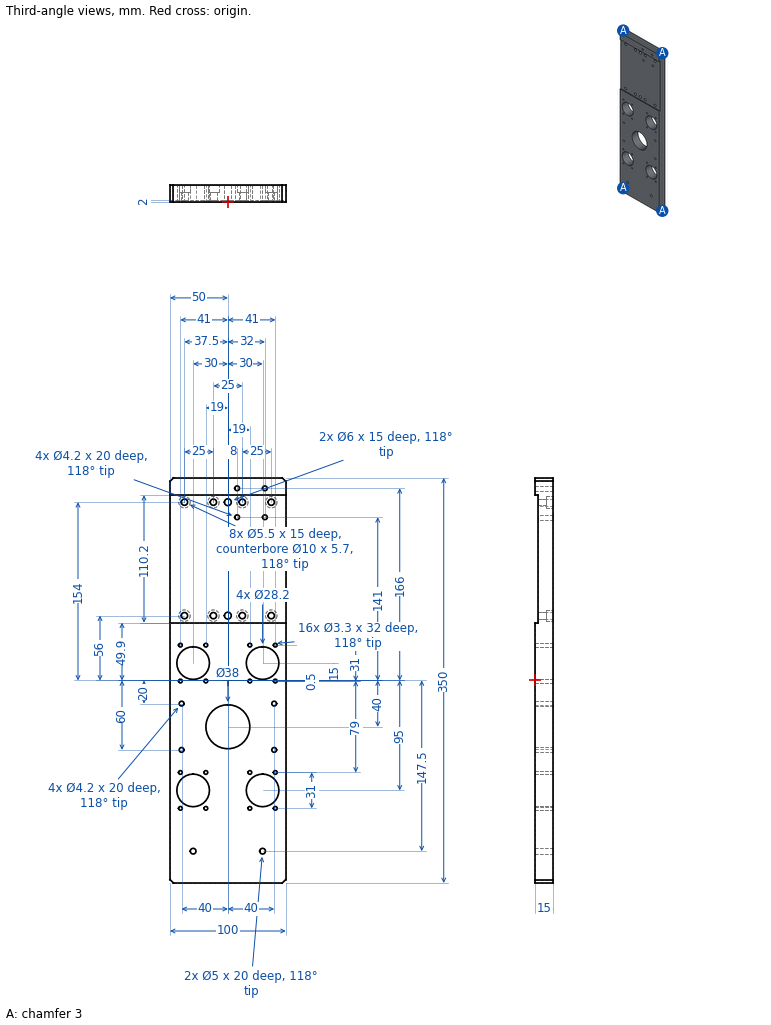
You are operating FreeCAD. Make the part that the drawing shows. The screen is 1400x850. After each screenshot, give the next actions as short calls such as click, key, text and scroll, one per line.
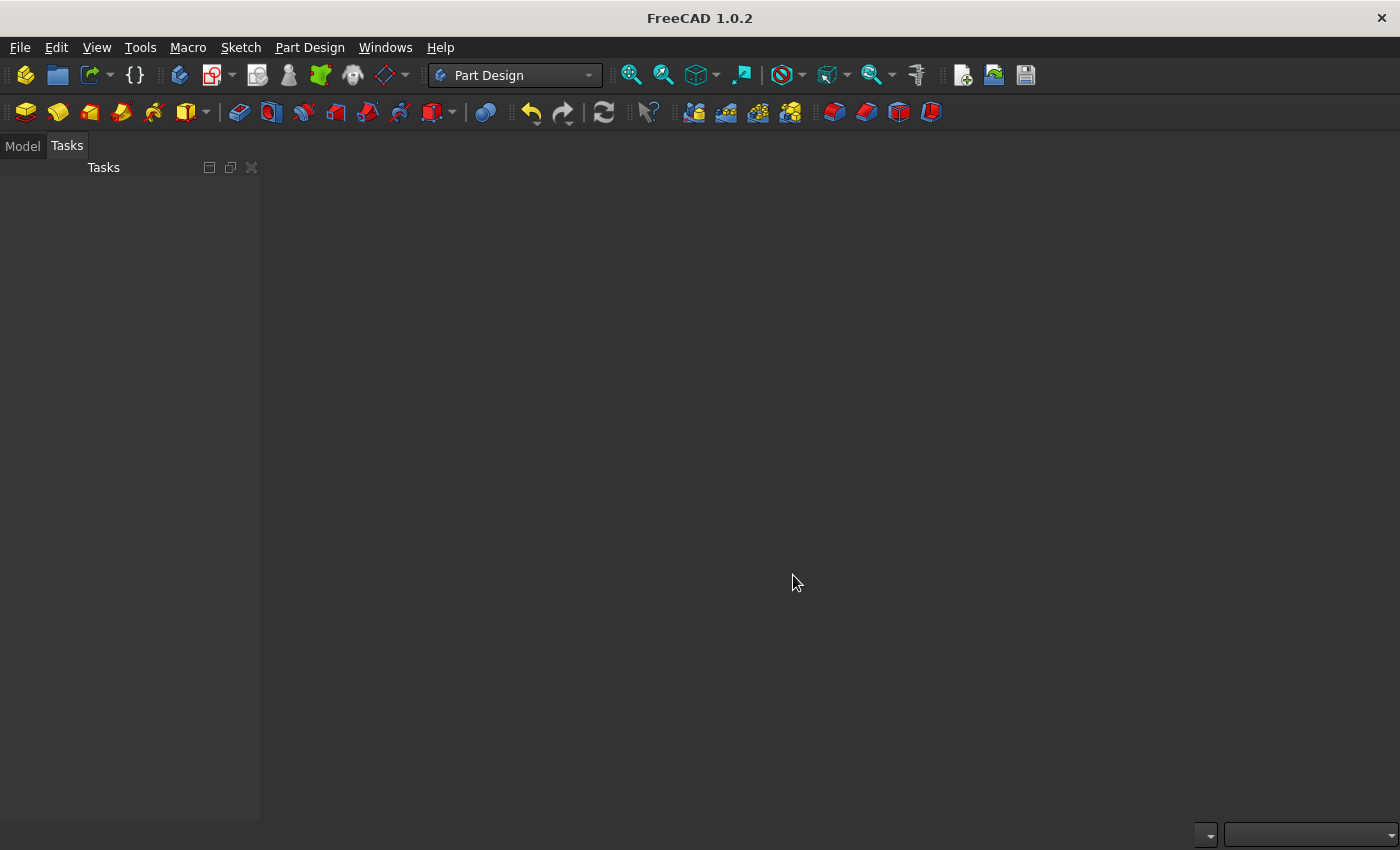
key(ctrl+n)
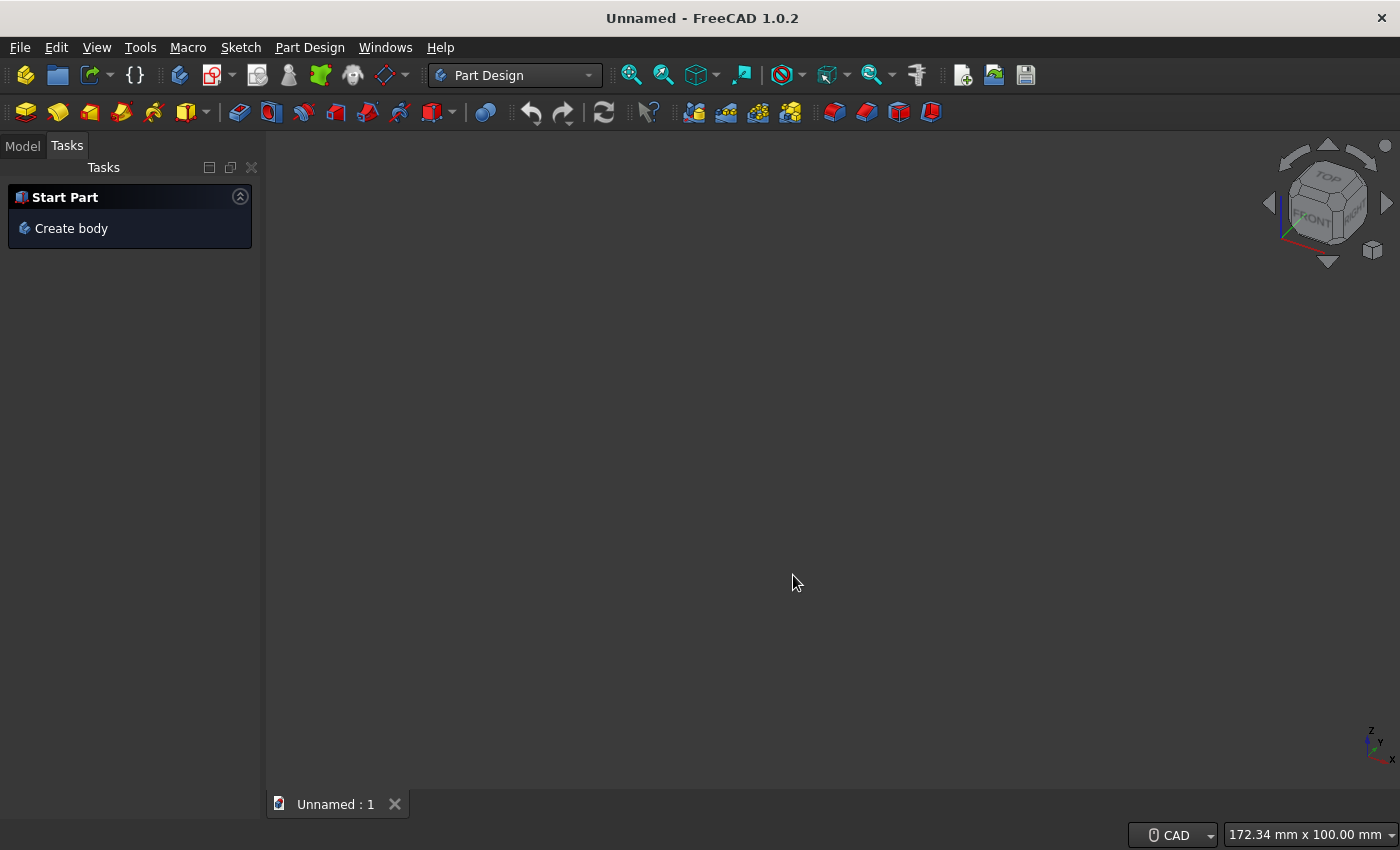
click(212, 76)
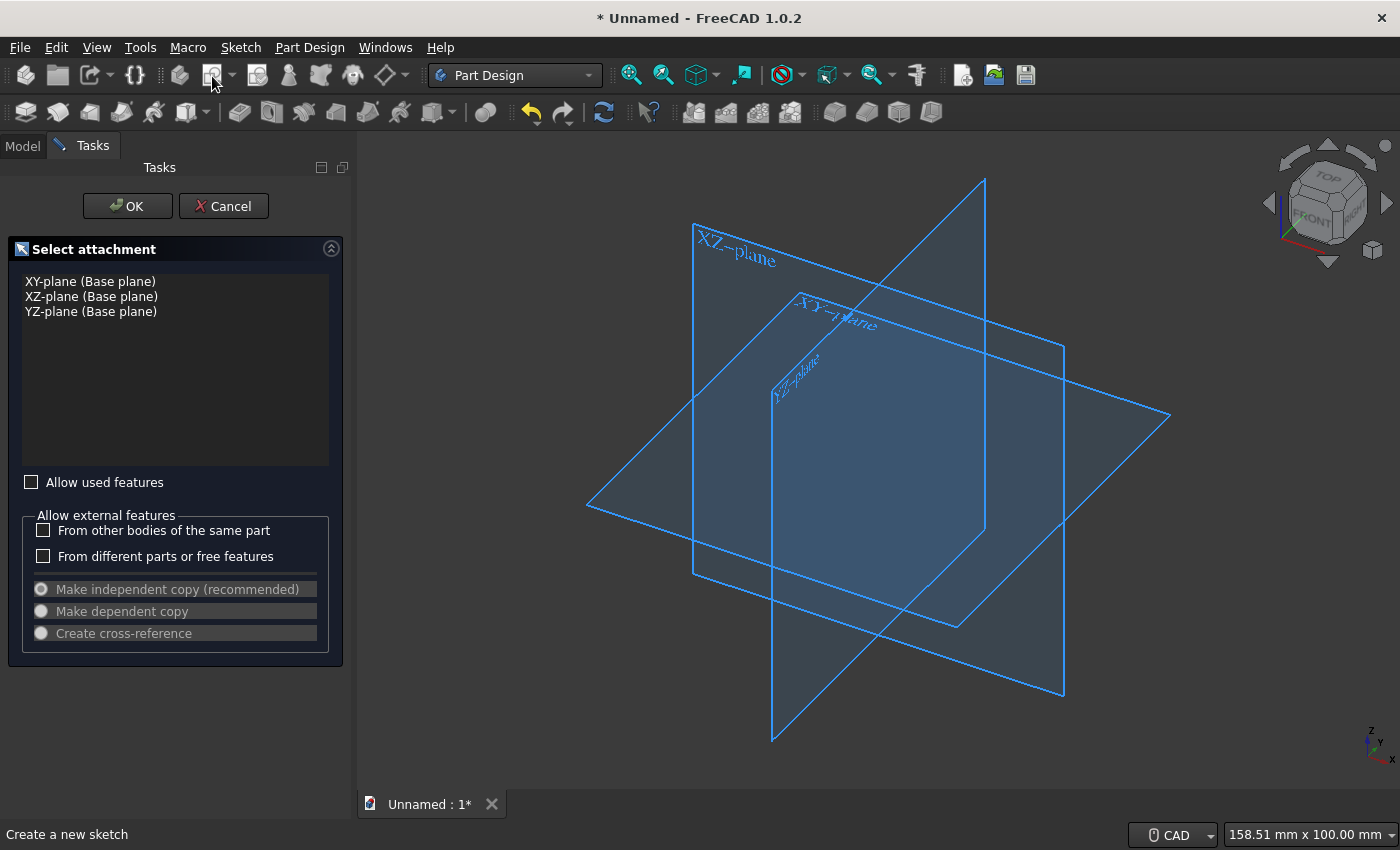
click(82, 296)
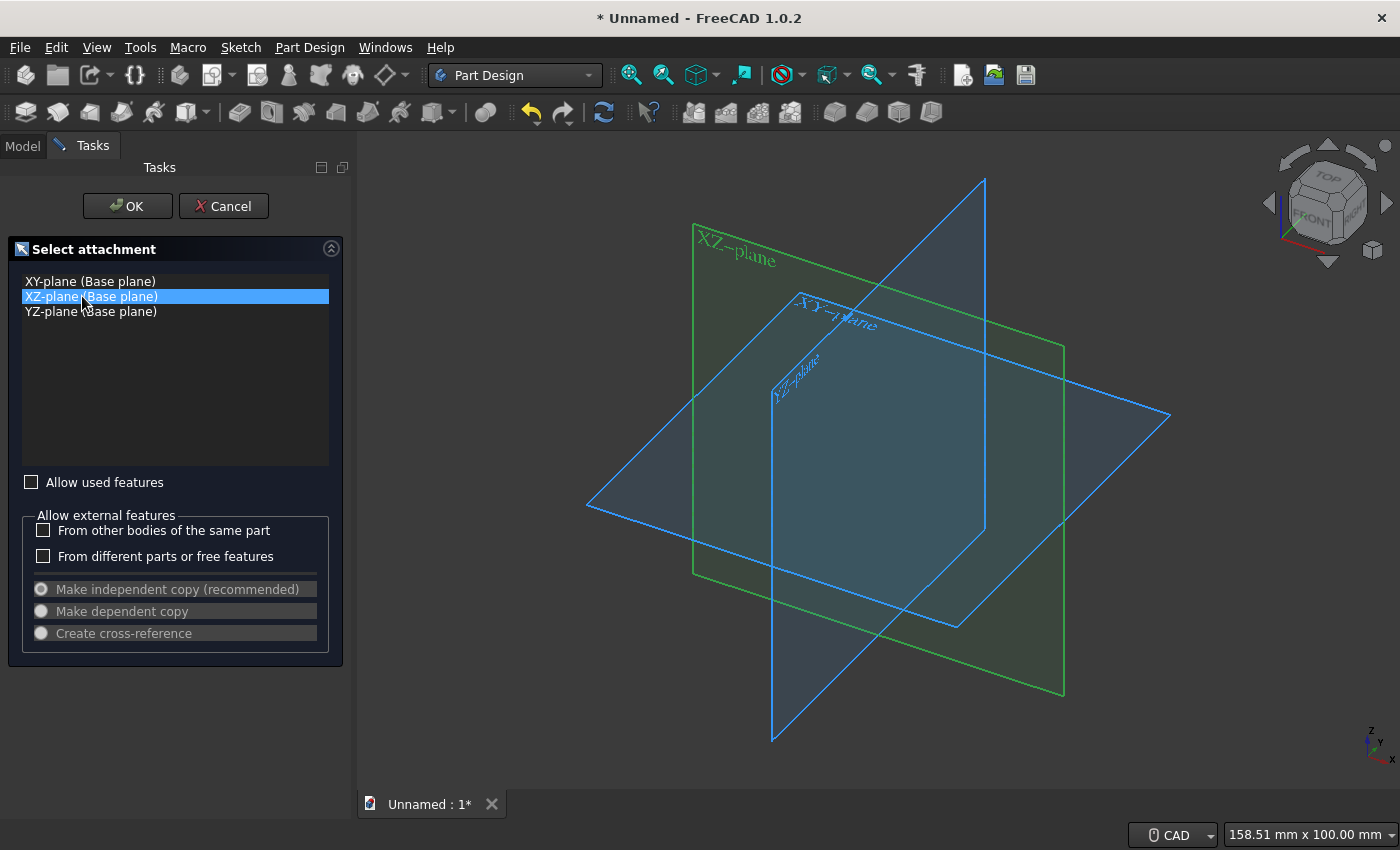
click(128, 206)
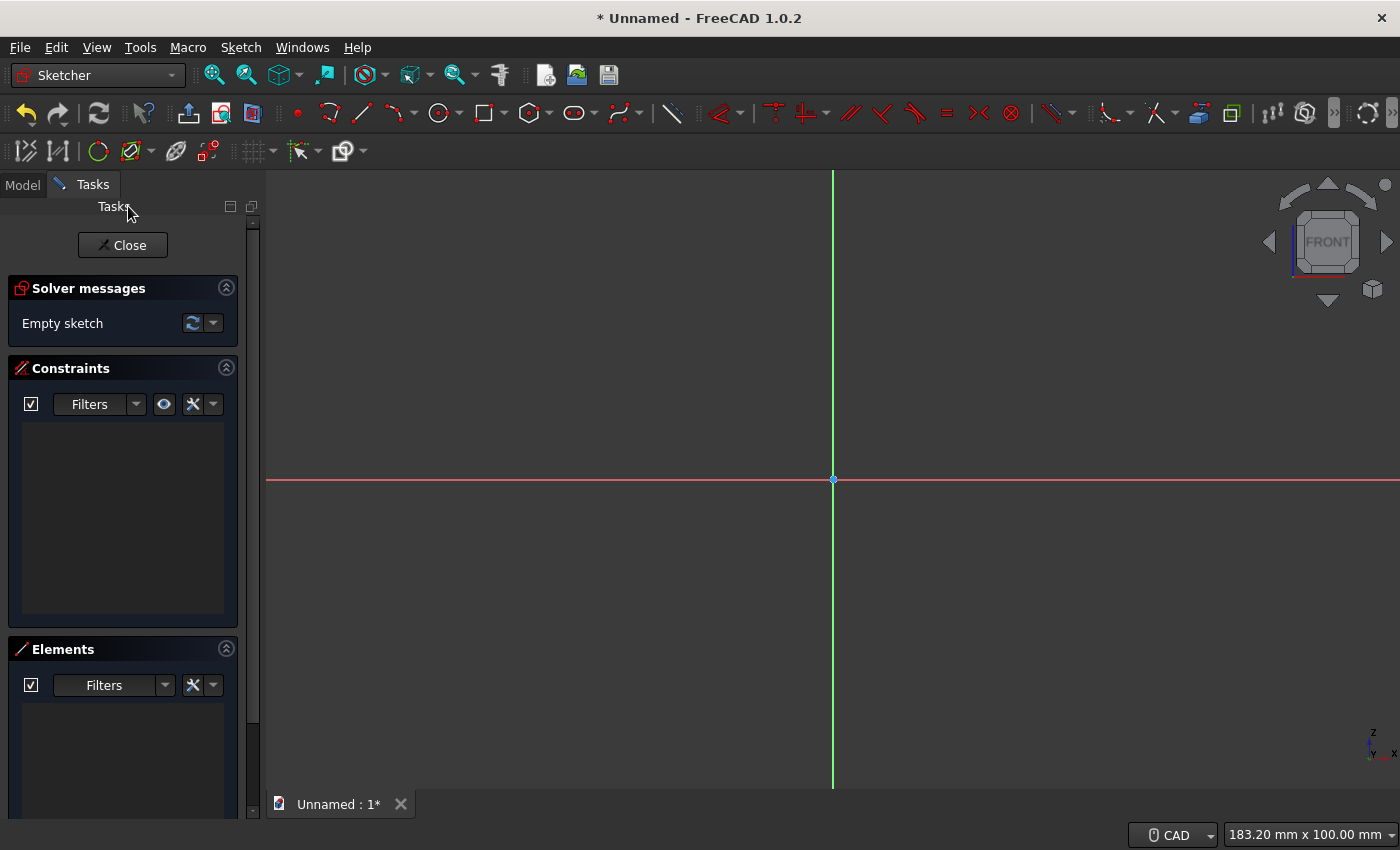
scroll(747, 480, down, 8)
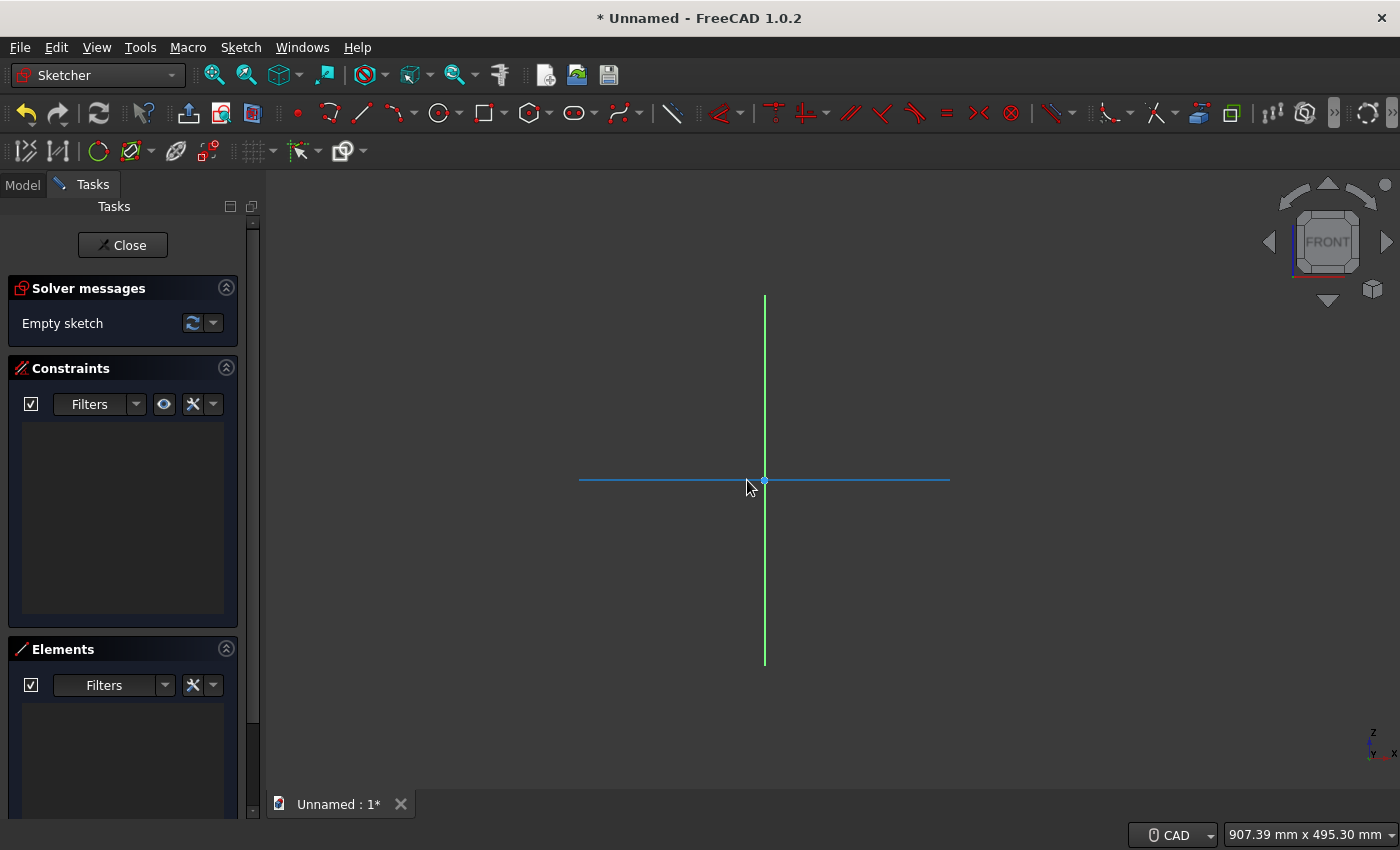
key(g)
key(v)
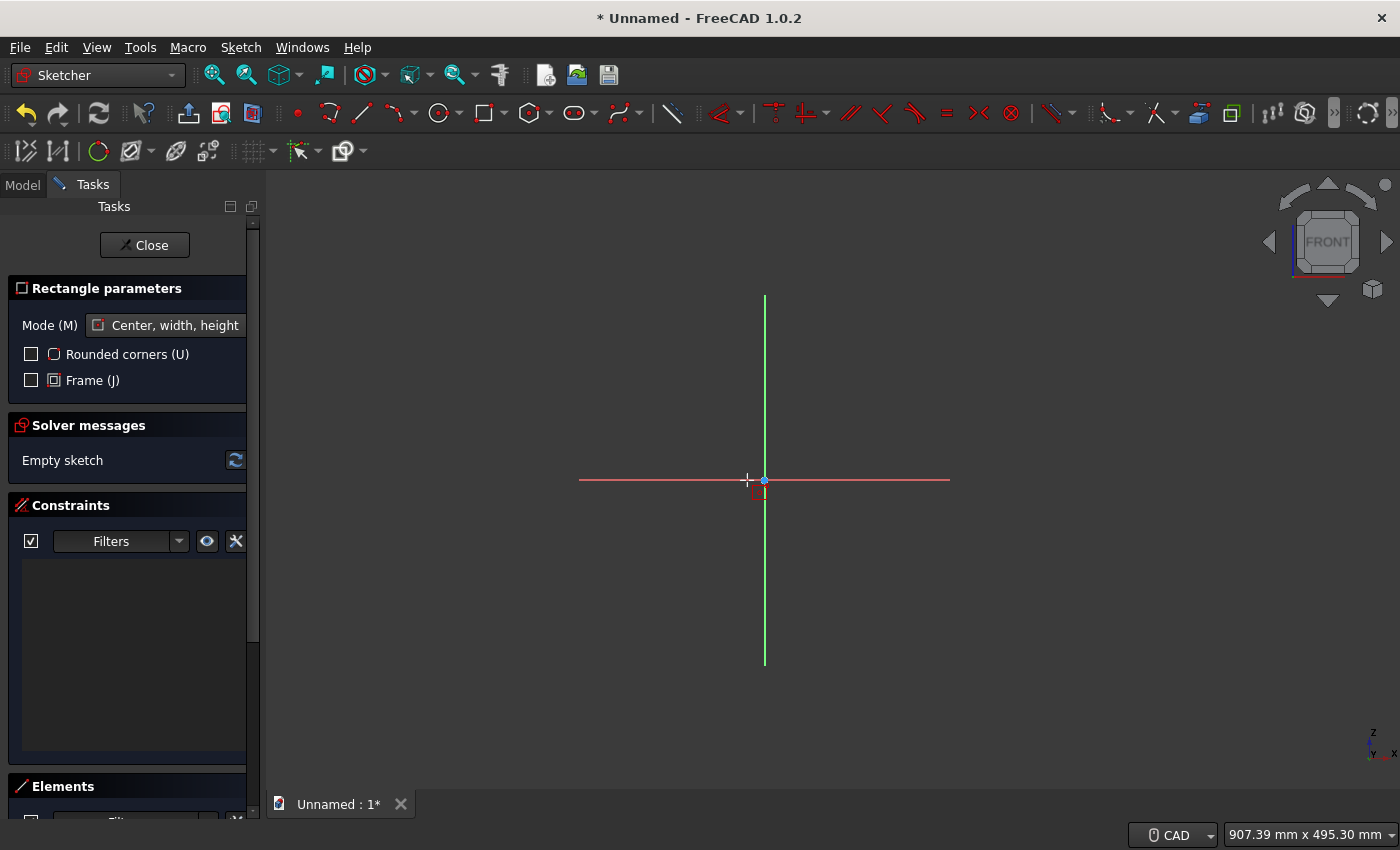
click(765, 480)
click(827, 262)
key(Escape)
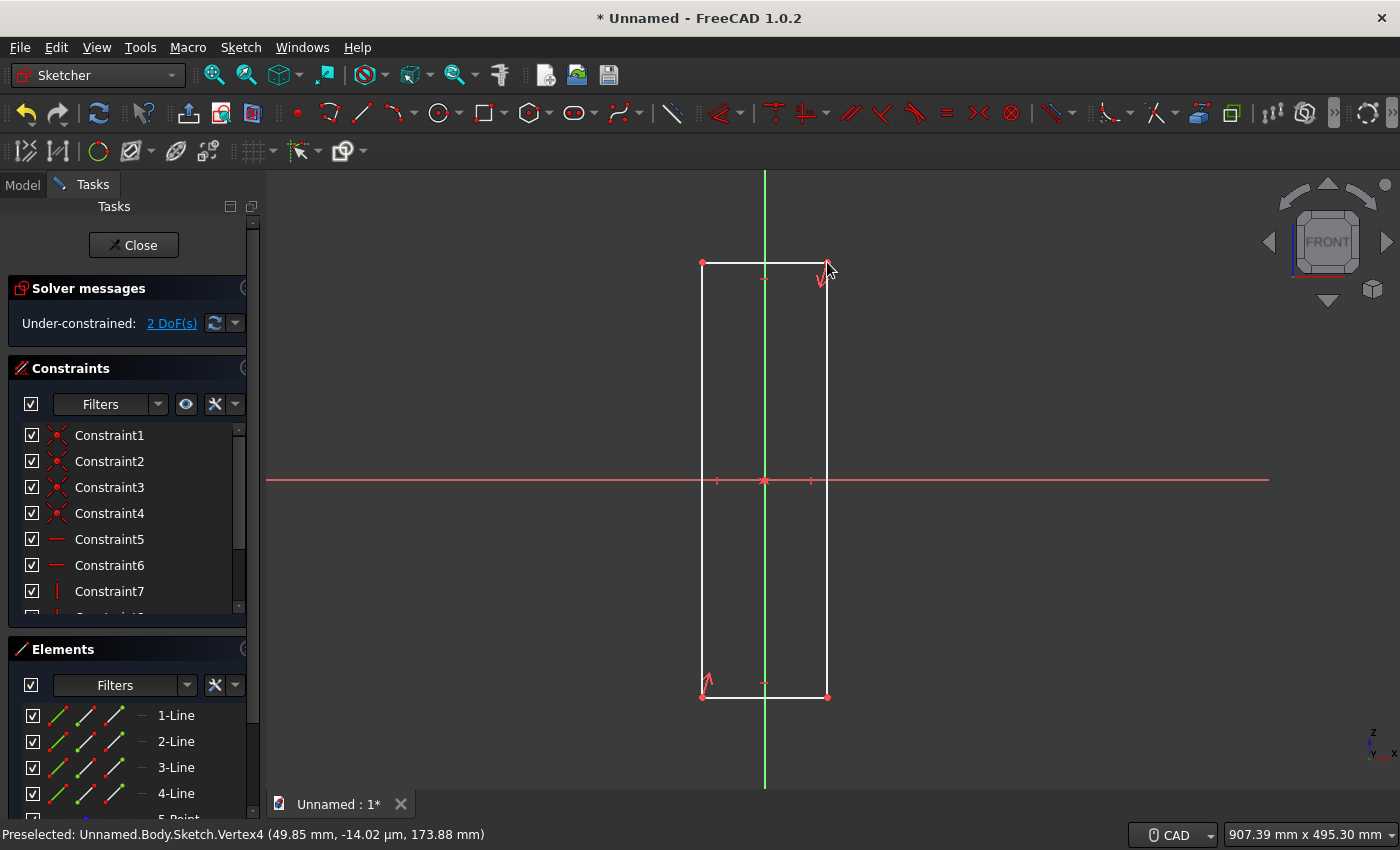
key(d)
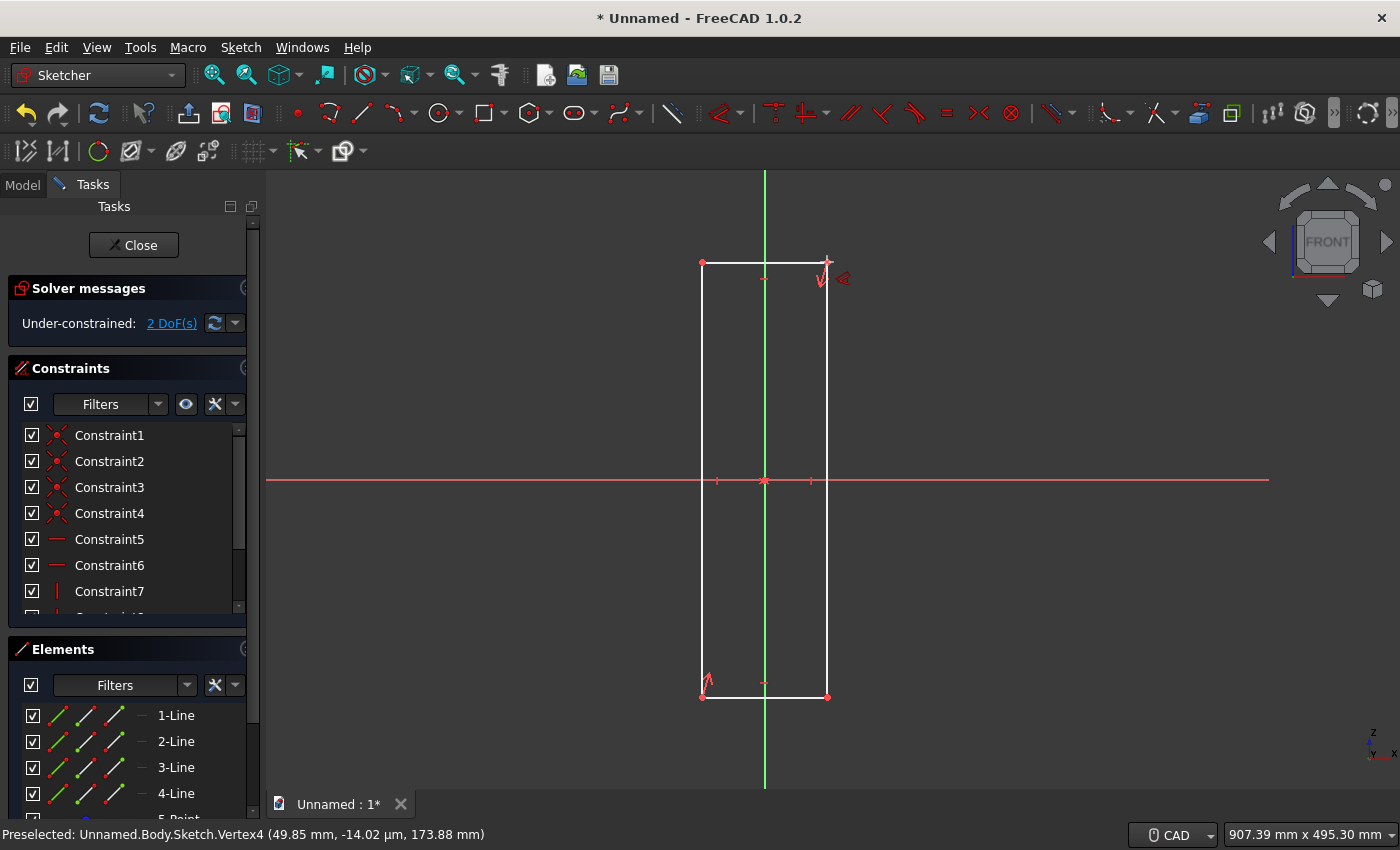
click(740, 698)
click(736, 732)